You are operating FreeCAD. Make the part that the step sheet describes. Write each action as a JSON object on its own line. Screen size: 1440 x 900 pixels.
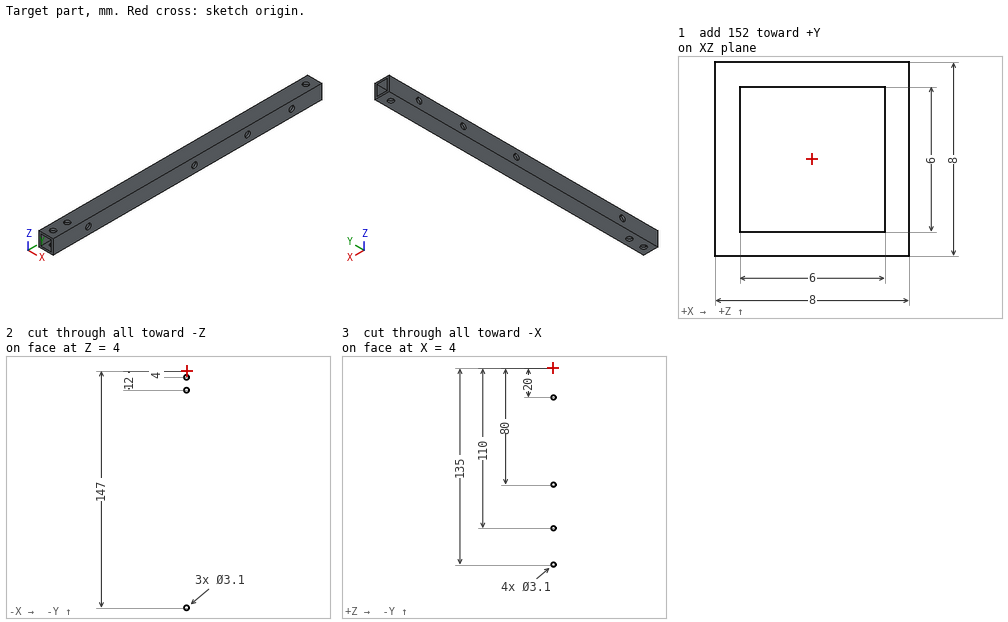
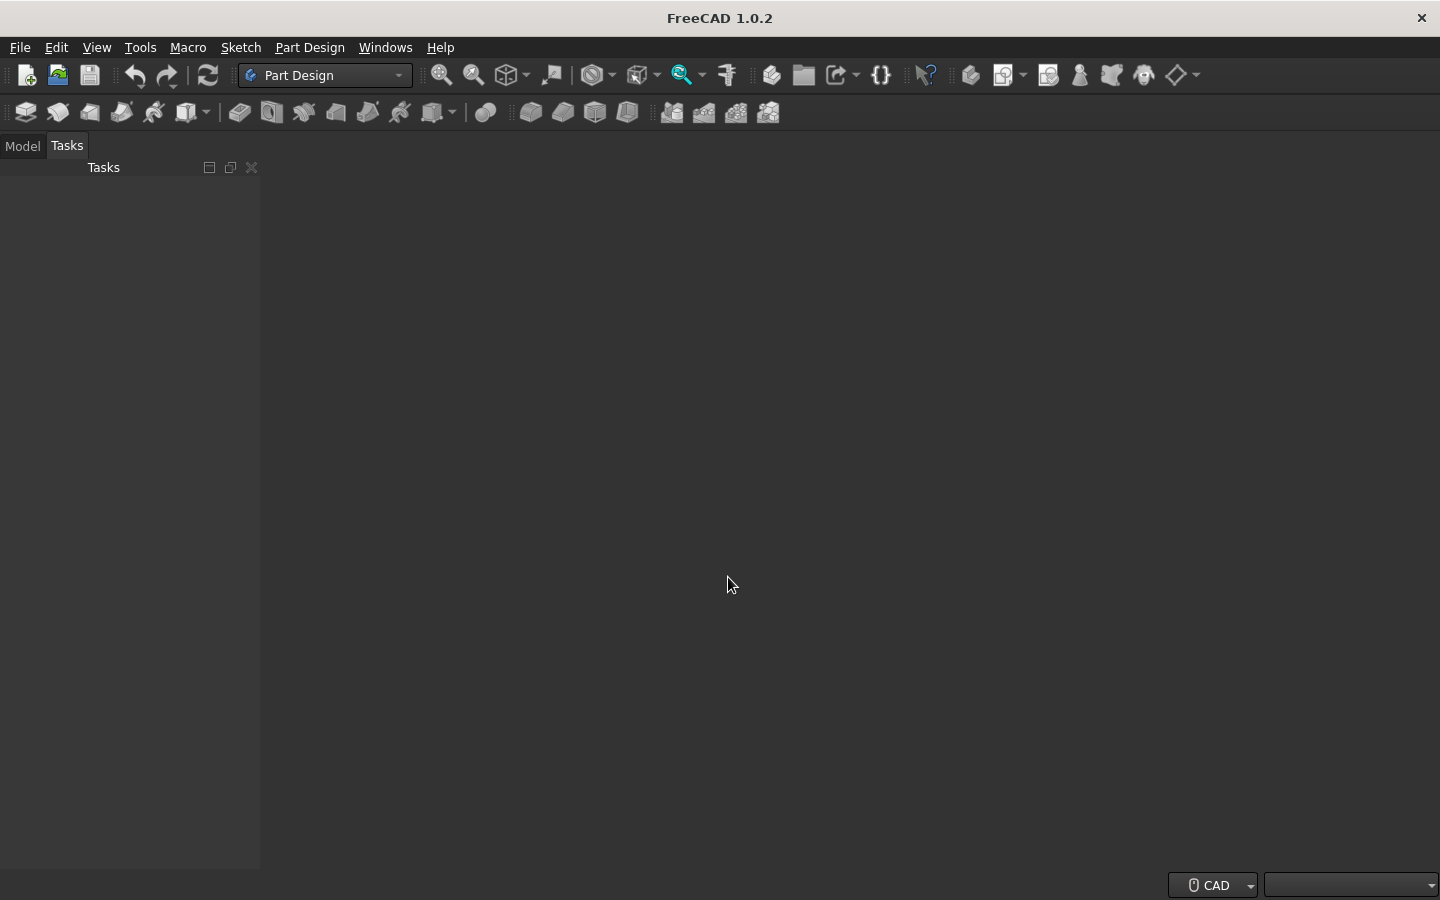
{"action": "left_click", "coordinate": [26, 76]}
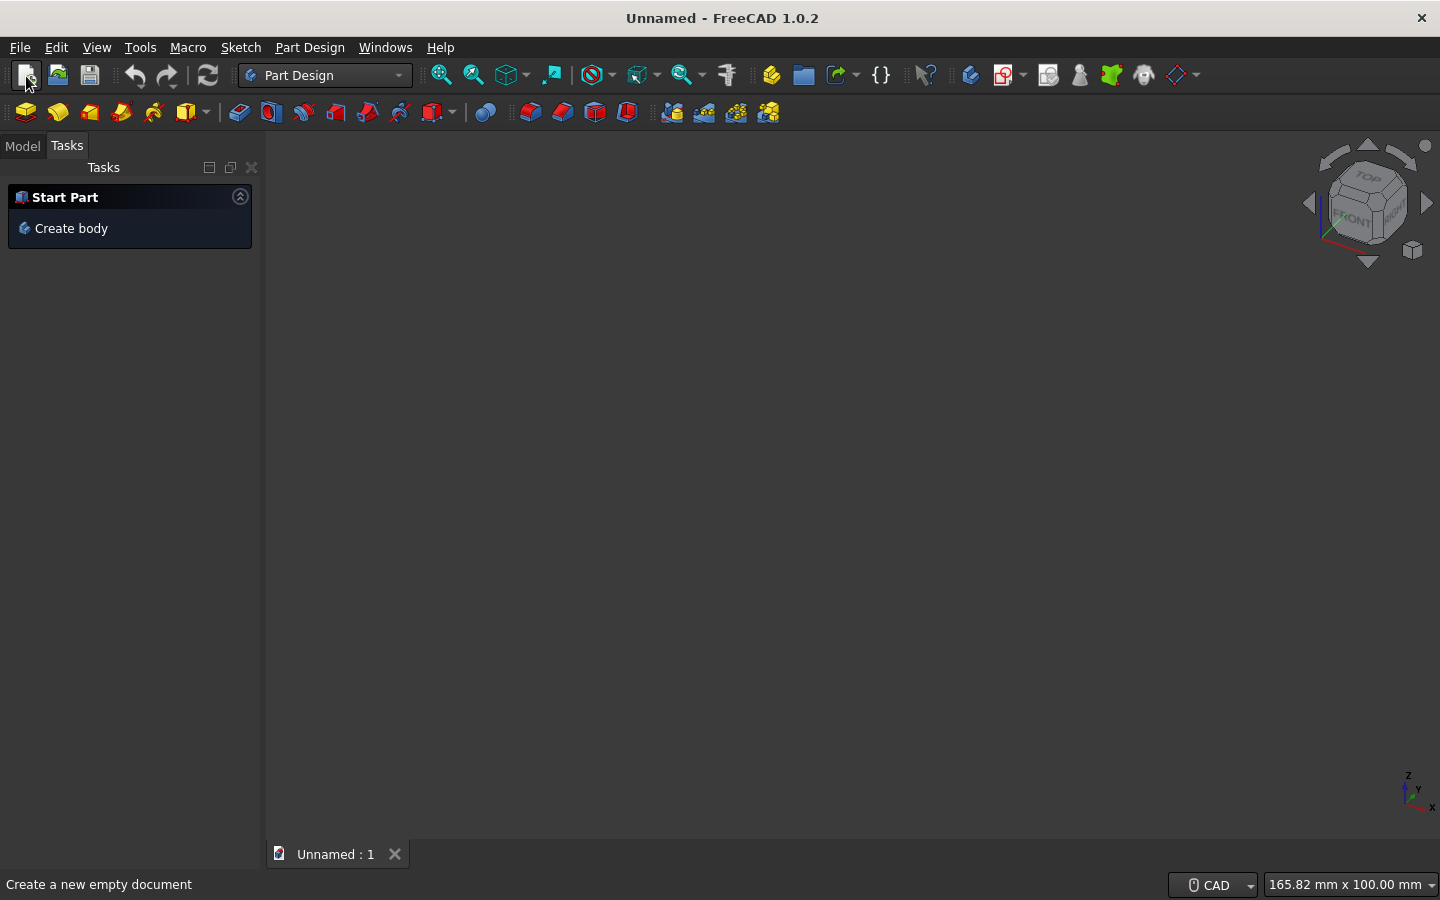
{"action": "left_click", "coordinate": [1004, 76]}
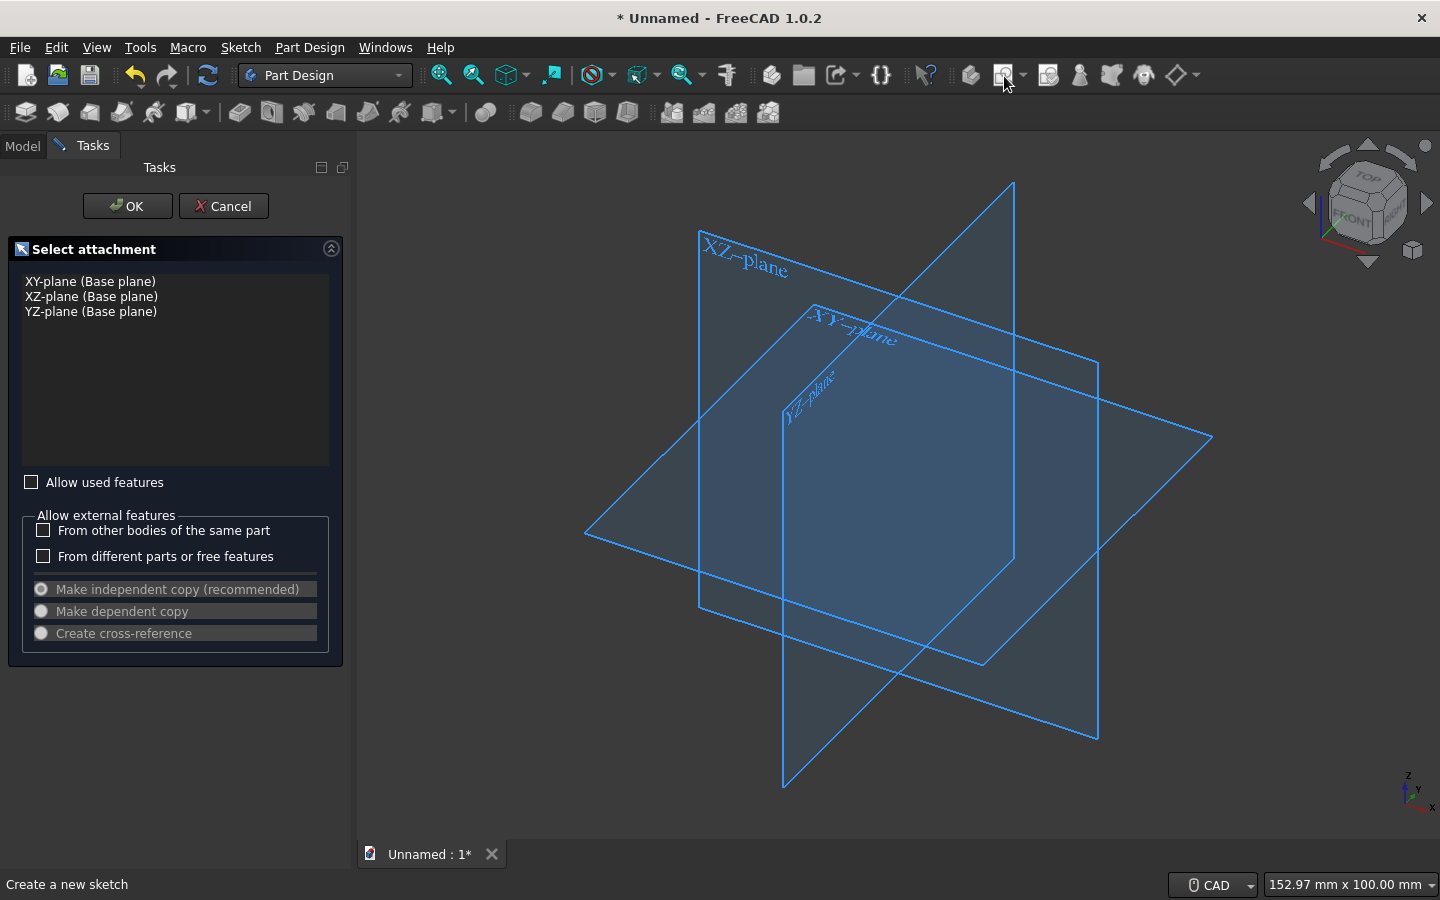
{"action": "left_click", "coordinate": [82, 296]}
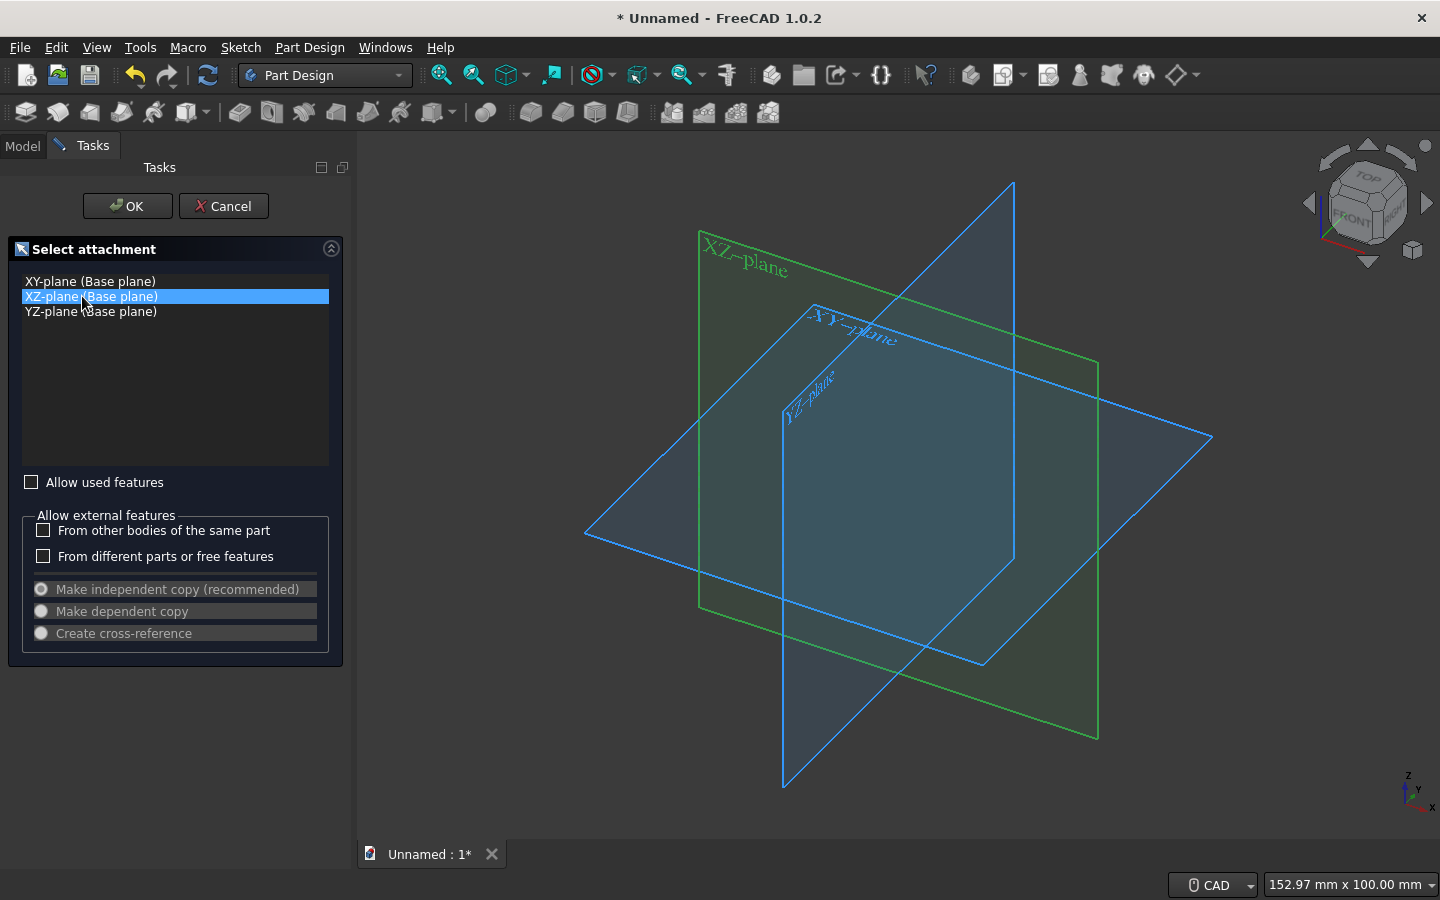
{"action": "left_click", "coordinate": [128, 206]}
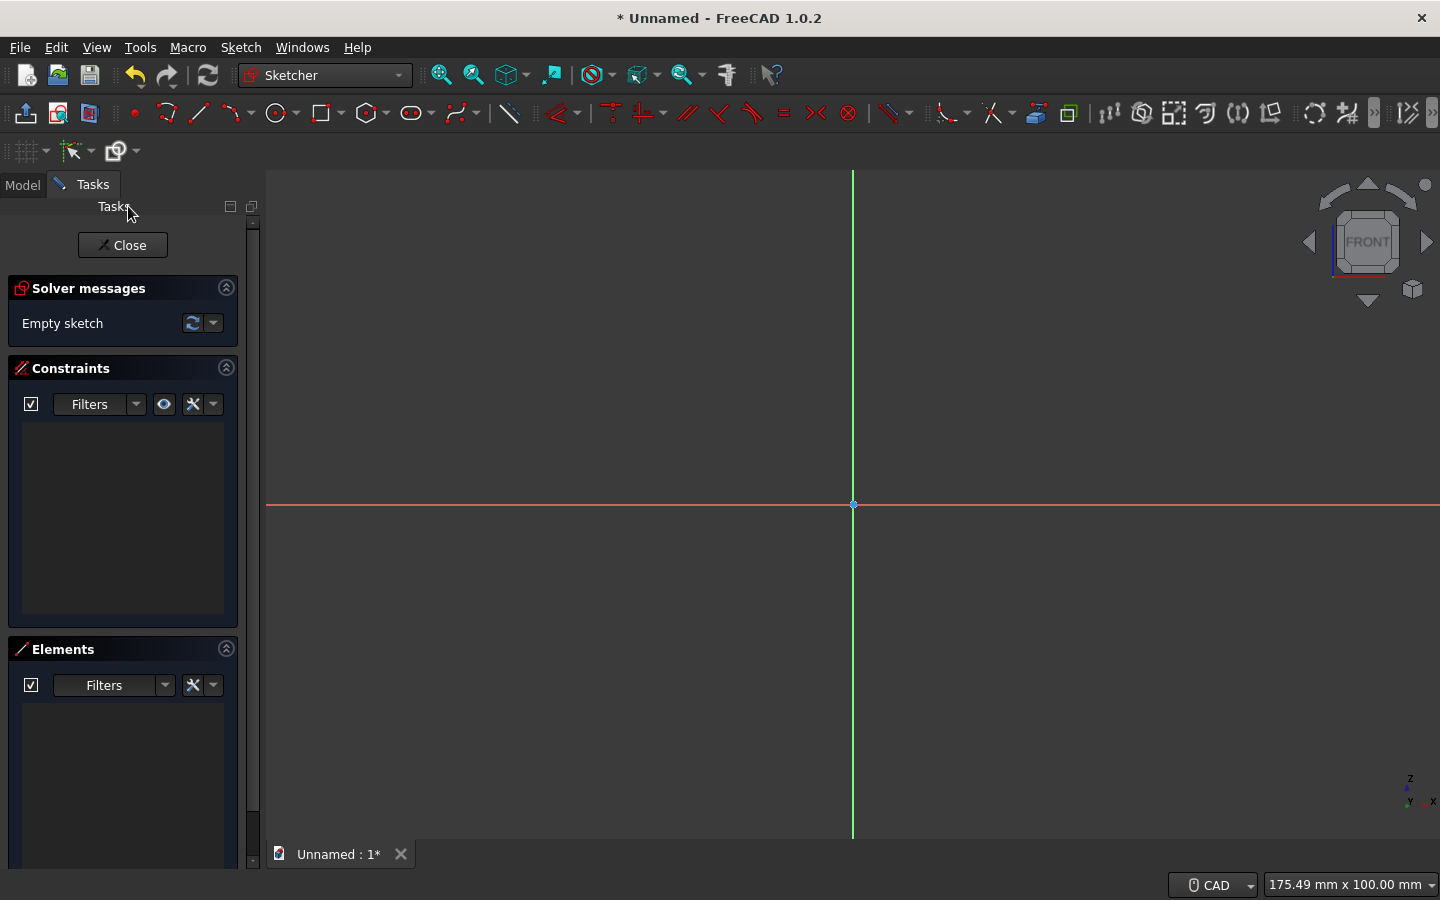
{"action": "scroll", "coordinate": [864, 504], "scroll_direction": "up", "scroll_amount": 10}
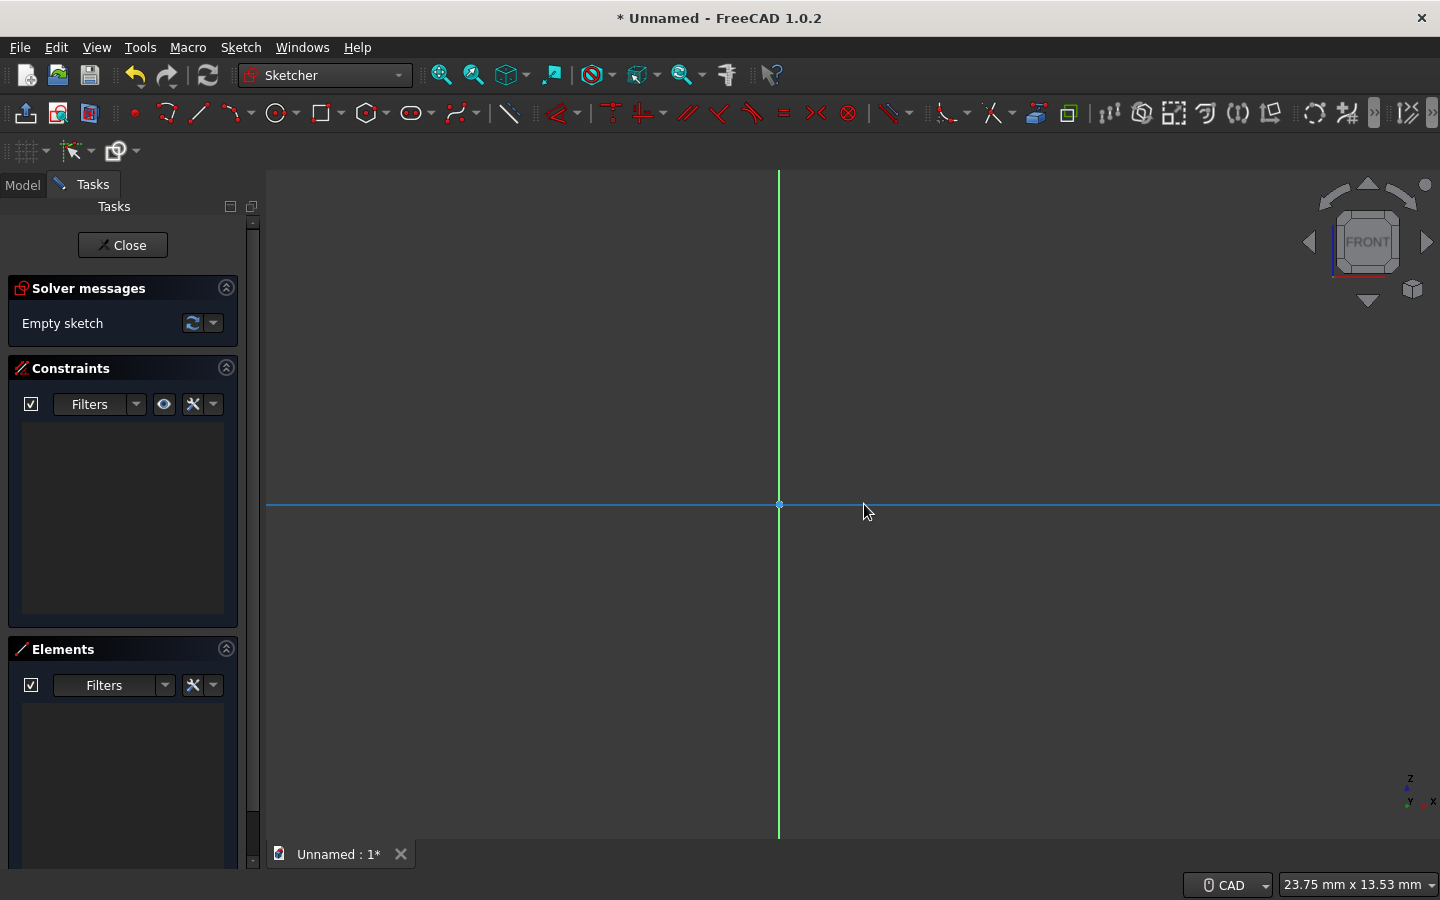
{"action": "left_click", "coordinate": [344, 114]}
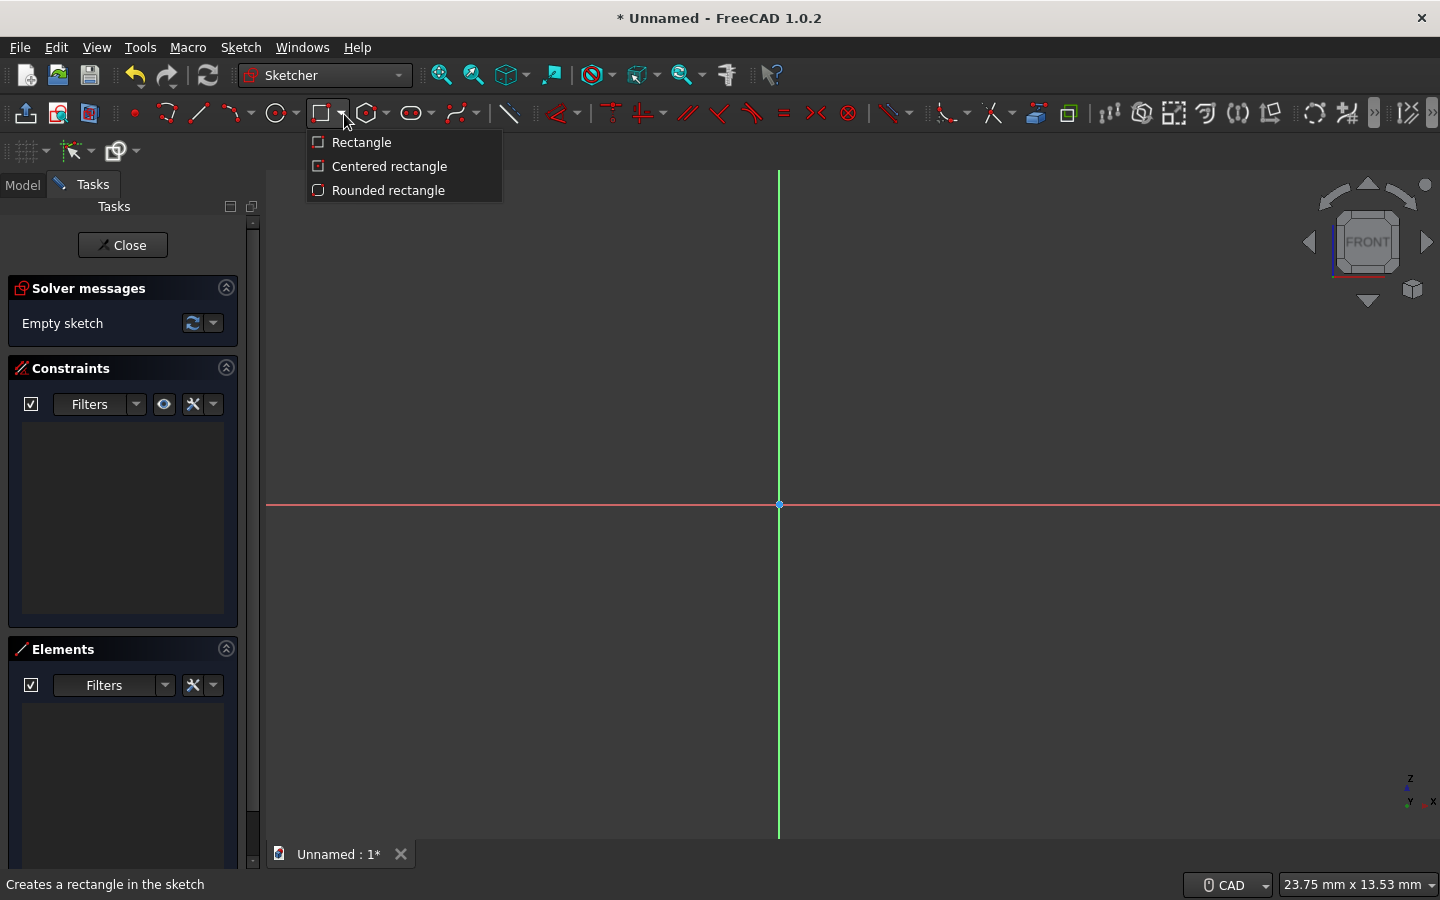
{"action": "left_click", "coordinate": [404, 166]}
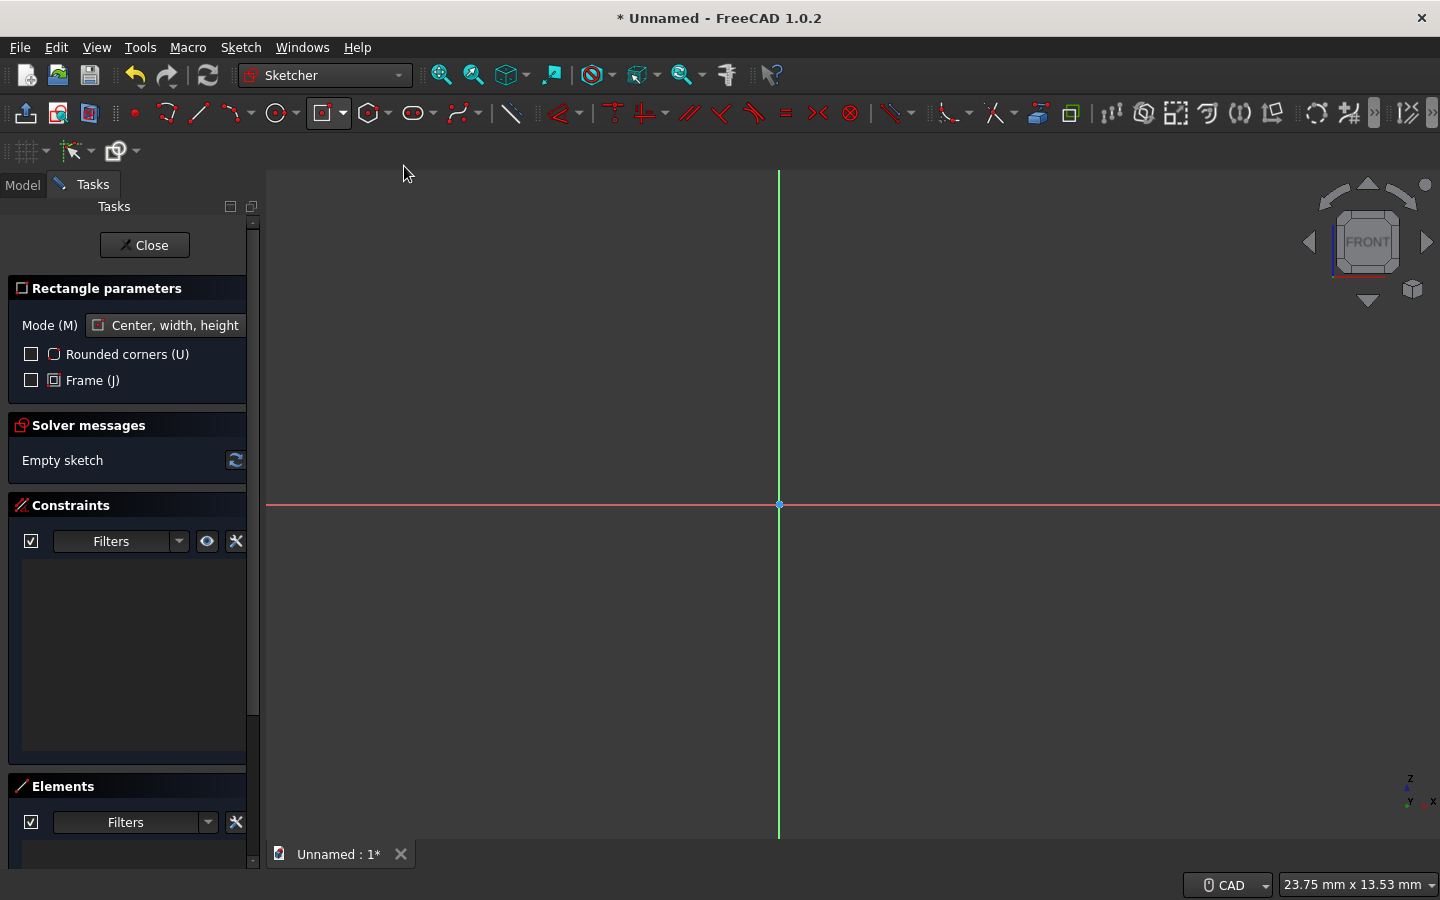
{"action": "left_click", "coordinate": [779, 504]}
{"action": "mouse_move", "coordinate": [977, 307]}